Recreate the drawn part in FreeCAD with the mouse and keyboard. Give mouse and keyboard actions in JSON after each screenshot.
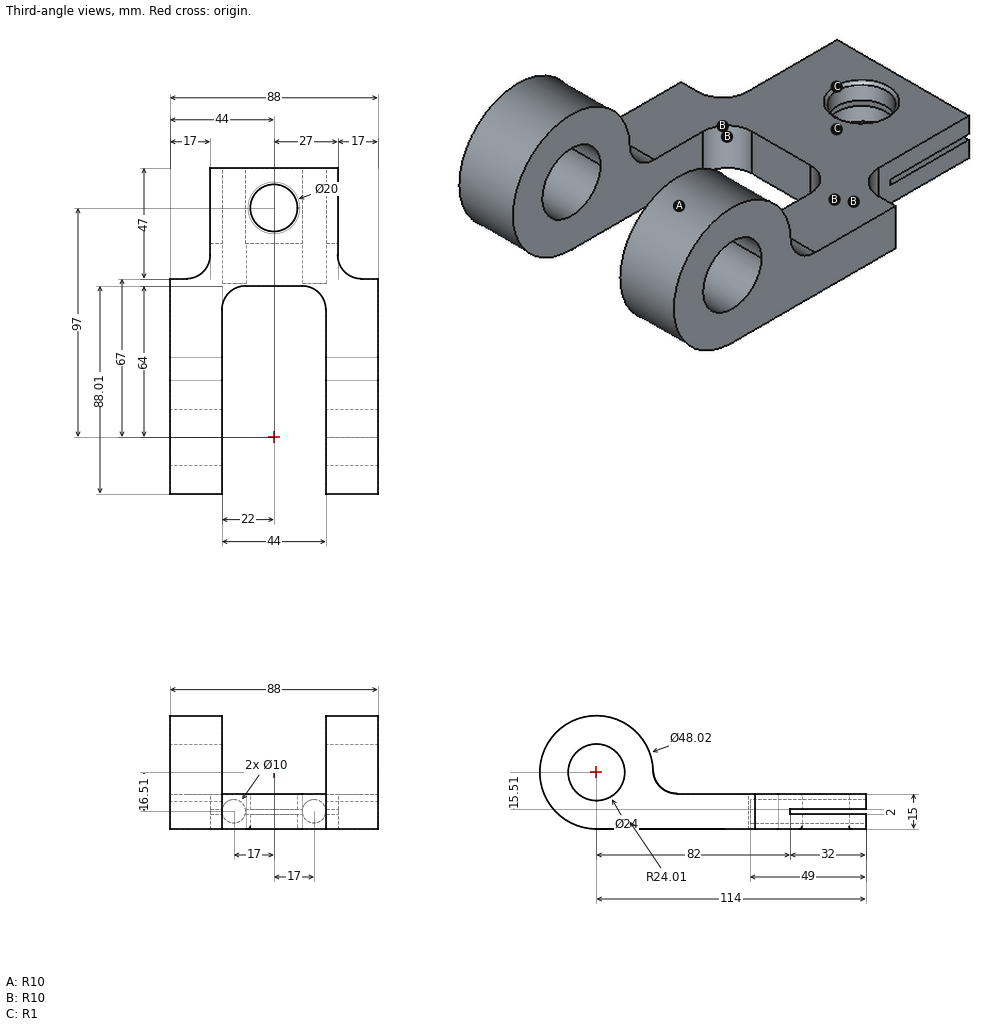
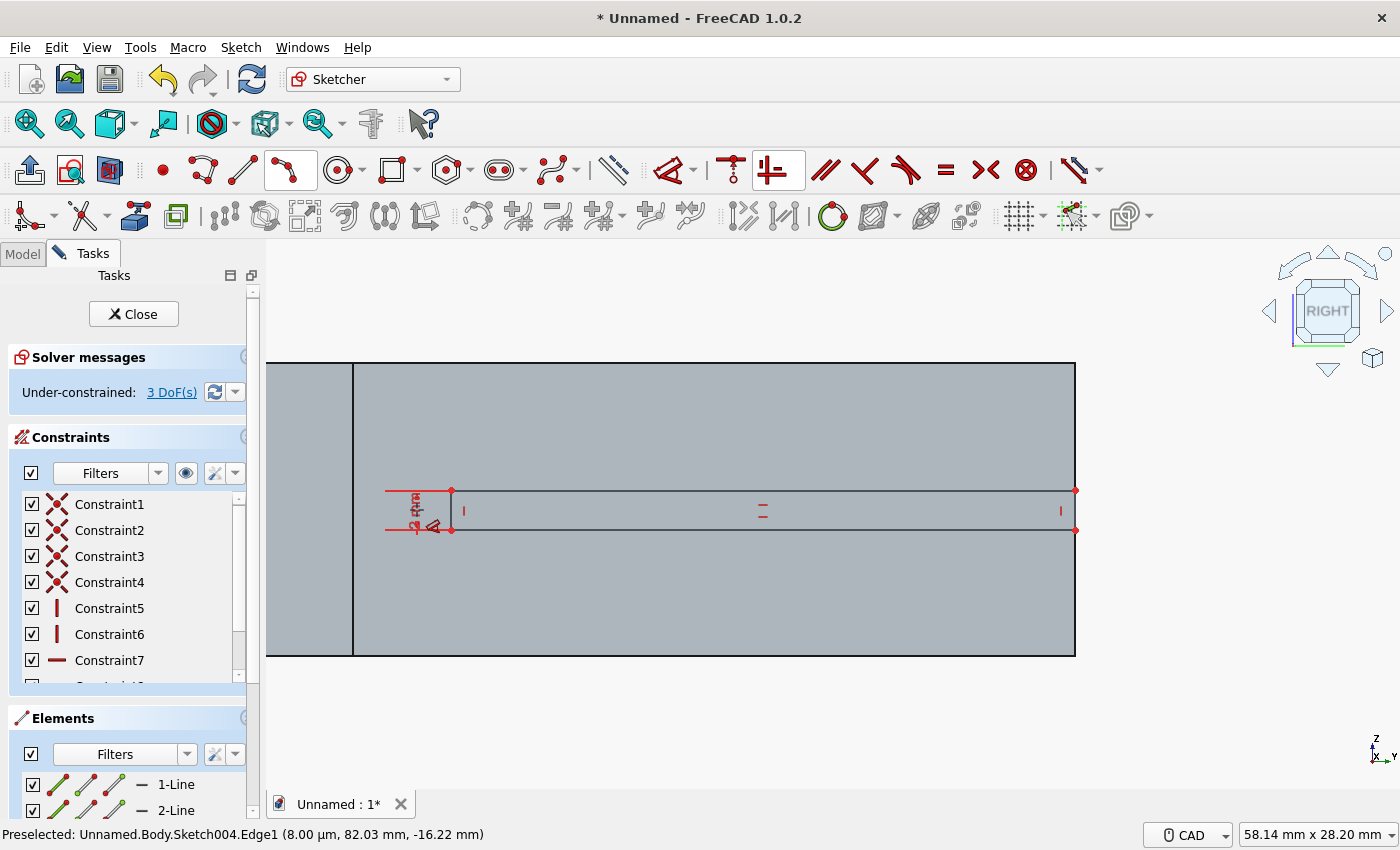
{"action": "left_click", "coordinate": [638, 530]}
{"action": "left_click", "coordinate": [763, 564]}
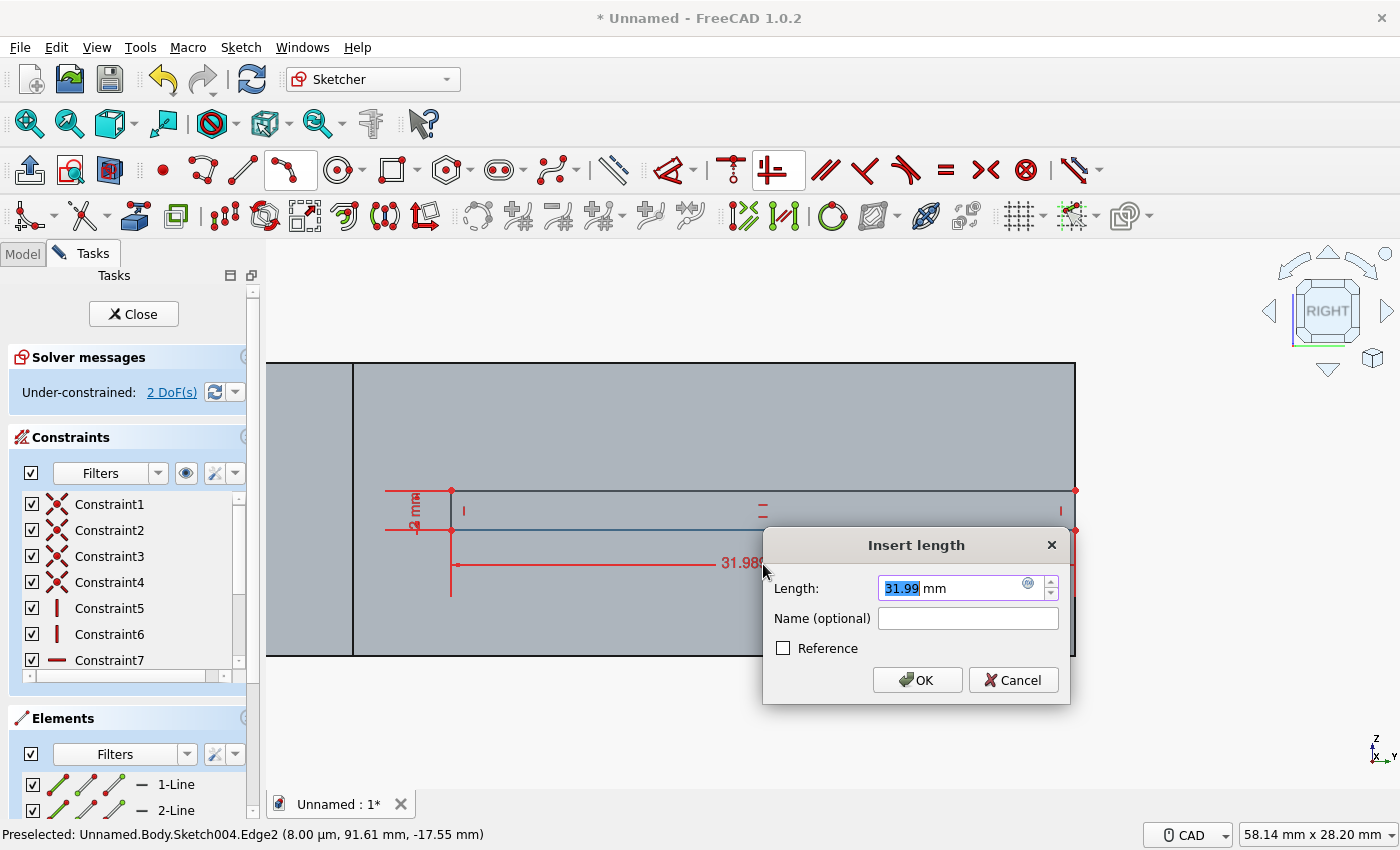
{"action": "type", "text": "32"}
{"action": "key", "text": "Return"}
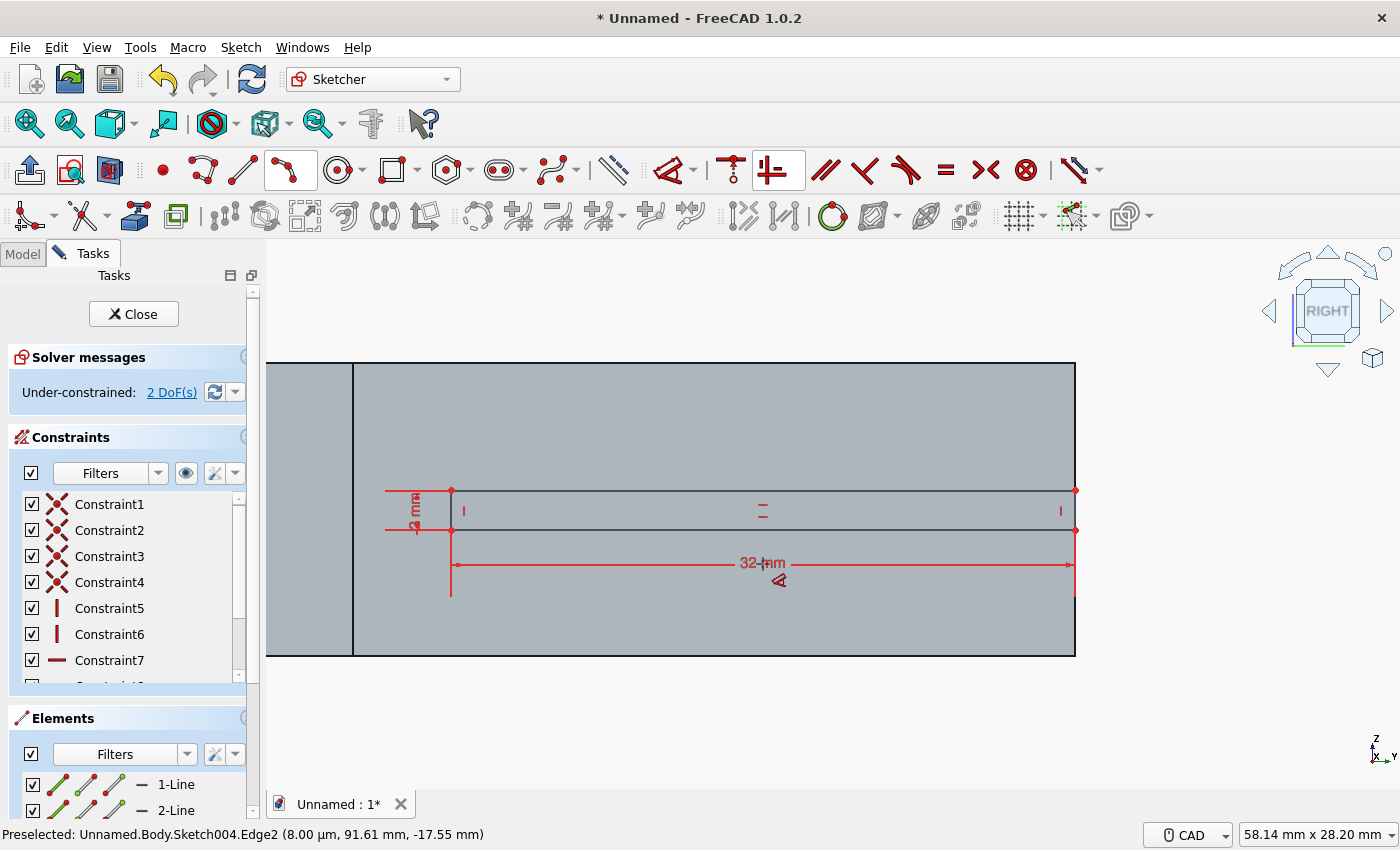
{"action": "left_click", "coordinate": [451, 491]}
{"action": "left_click", "coordinate": [336, 525]}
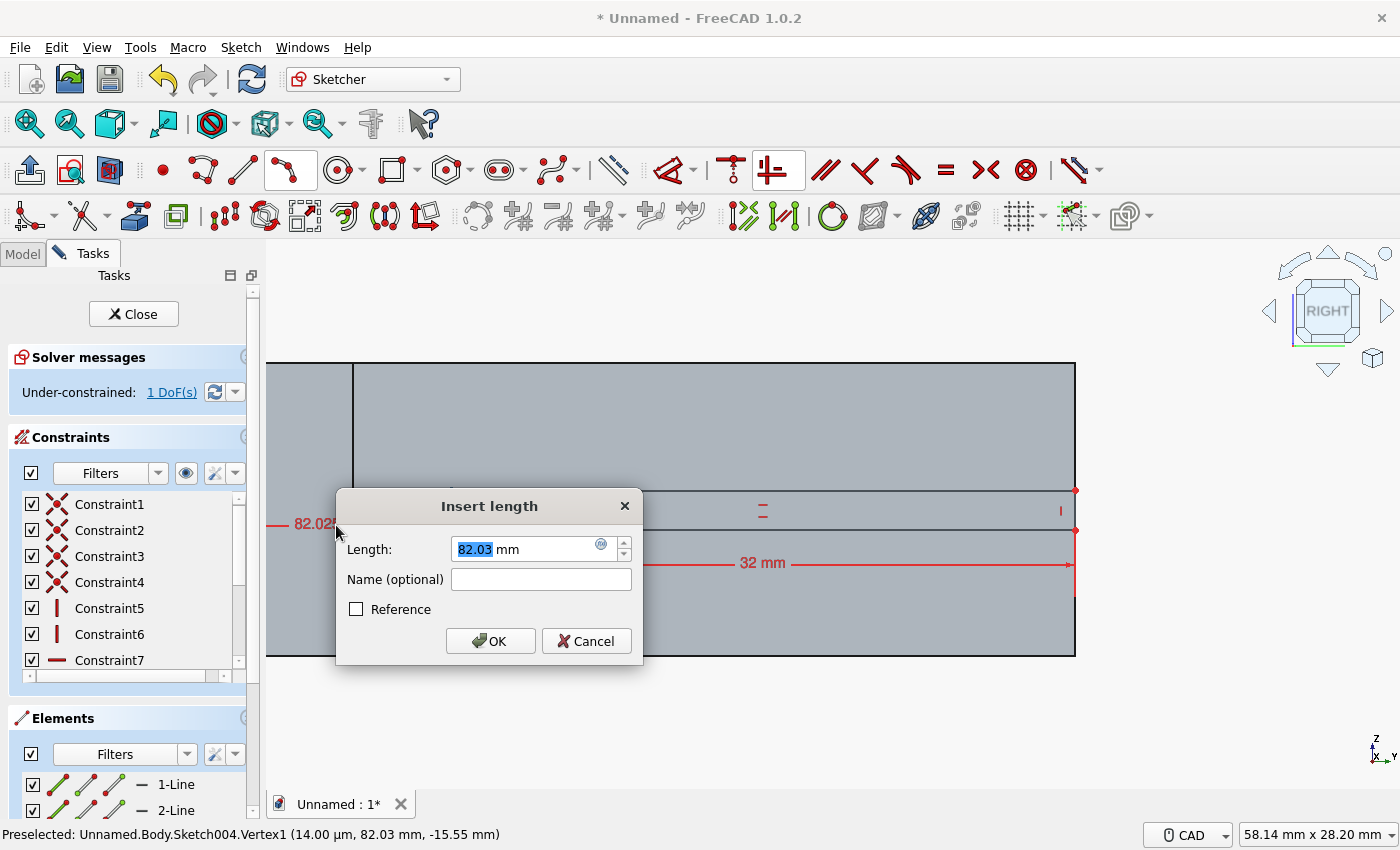
{"action": "type", "text": "82"}
{"action": "key", "text": "Return"}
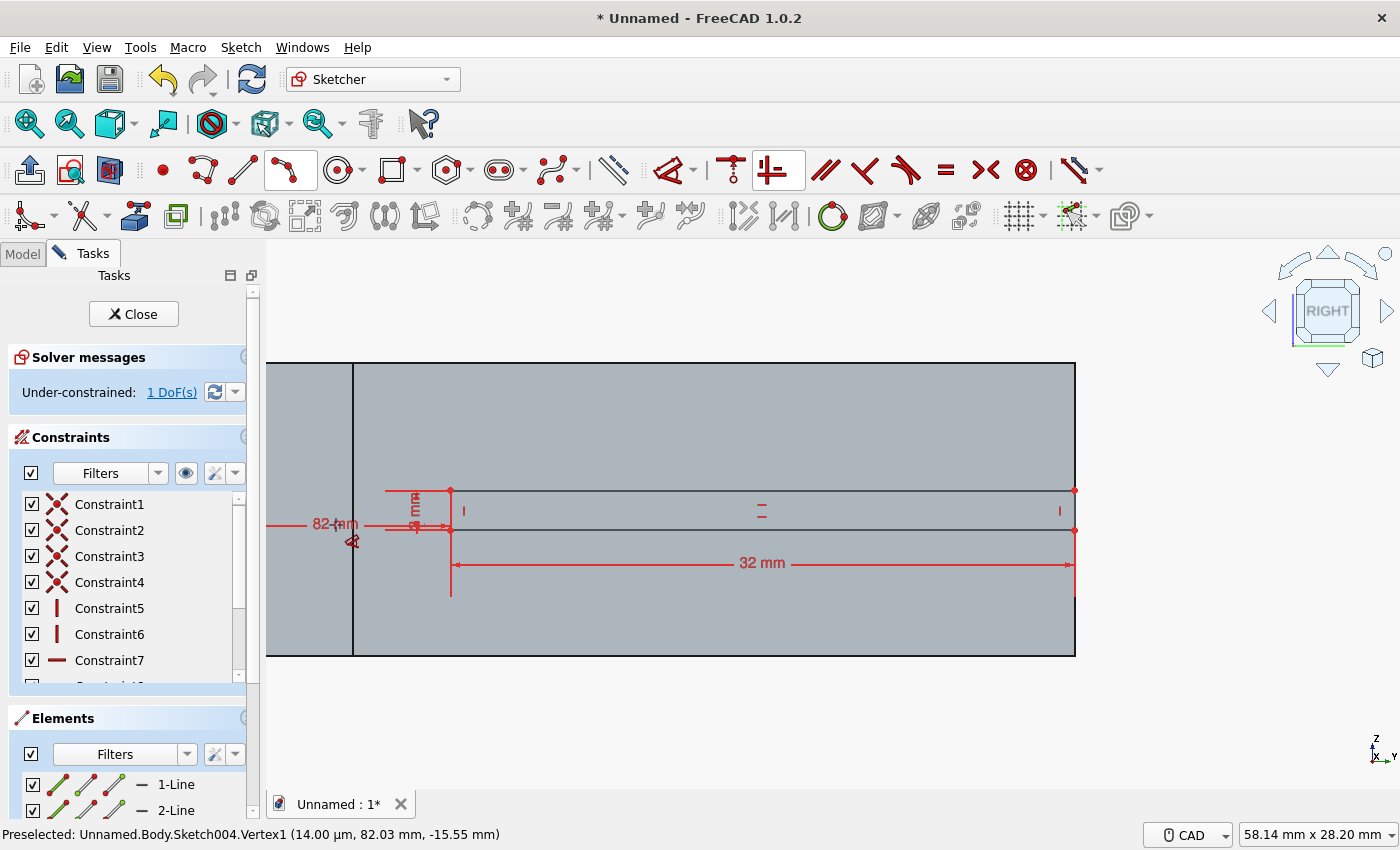
{"action": "left_click", "coordinate": [451, 491]}
{"action": "left_click", "coordinate": [485, 379]}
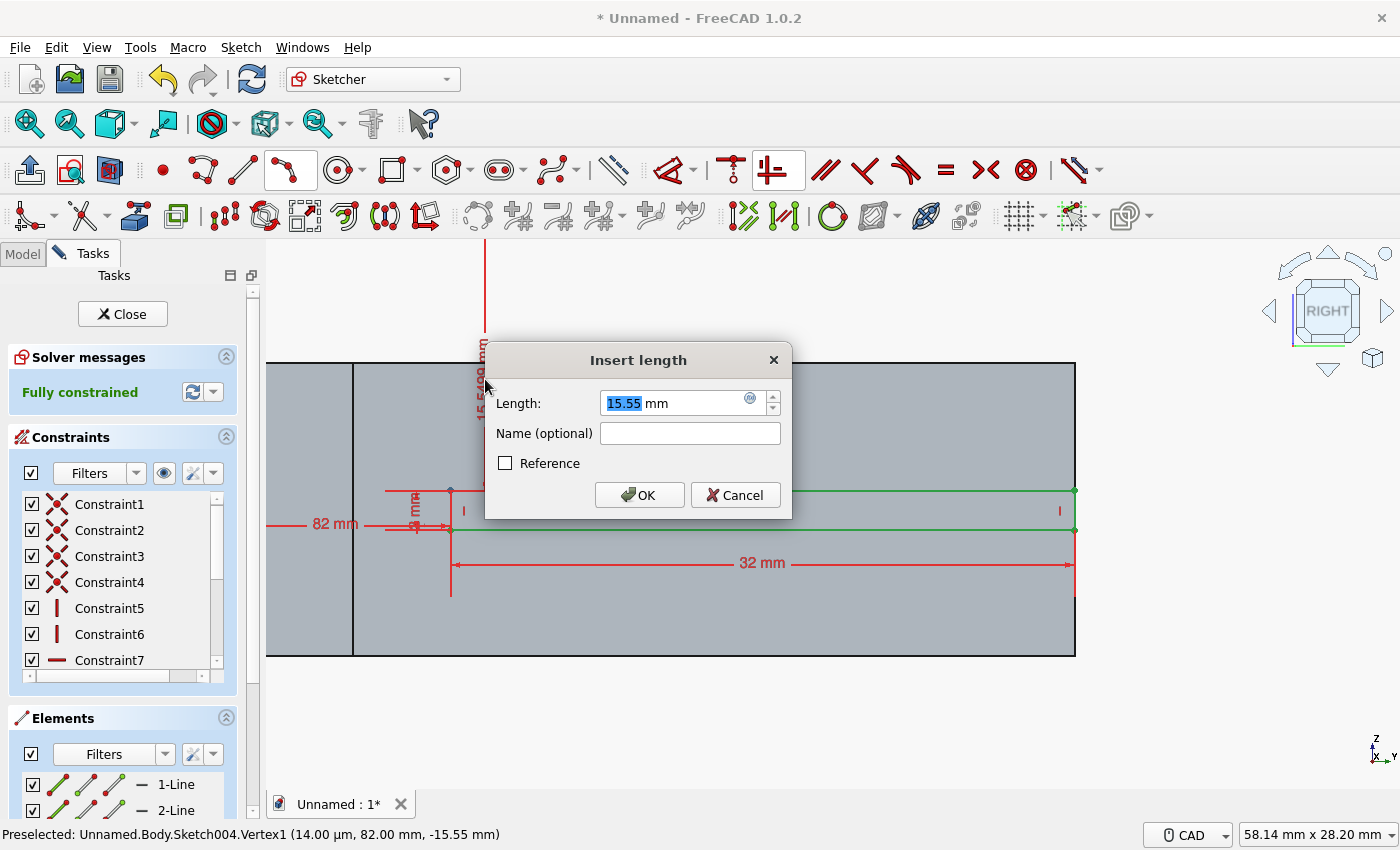
{"action": "type", "text": "15.51"}
{"action": "key", "text": "Return"}
{"action": "key", "text": "Escape"}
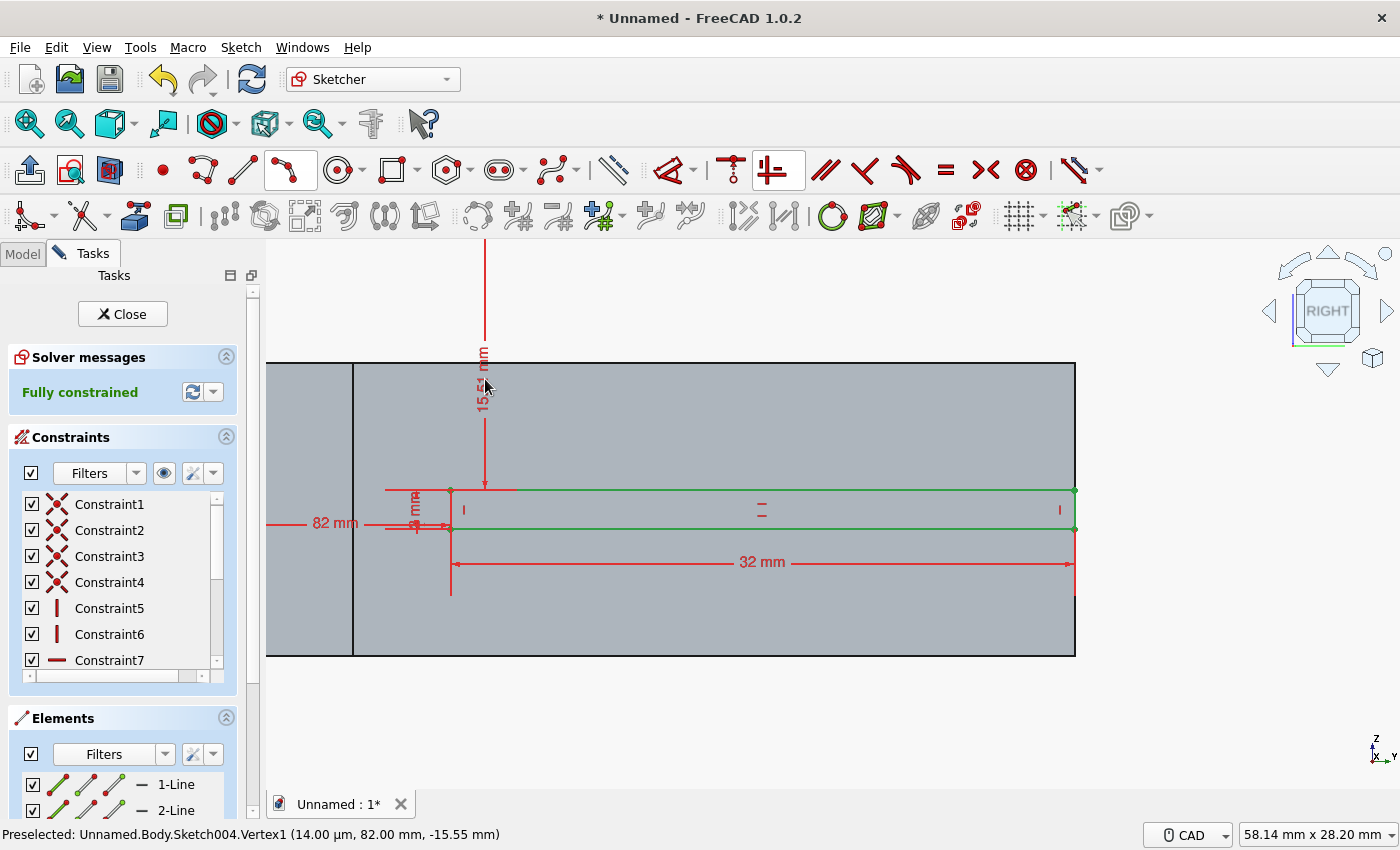
{"action": "left_click", "coordinate": [123, 314]}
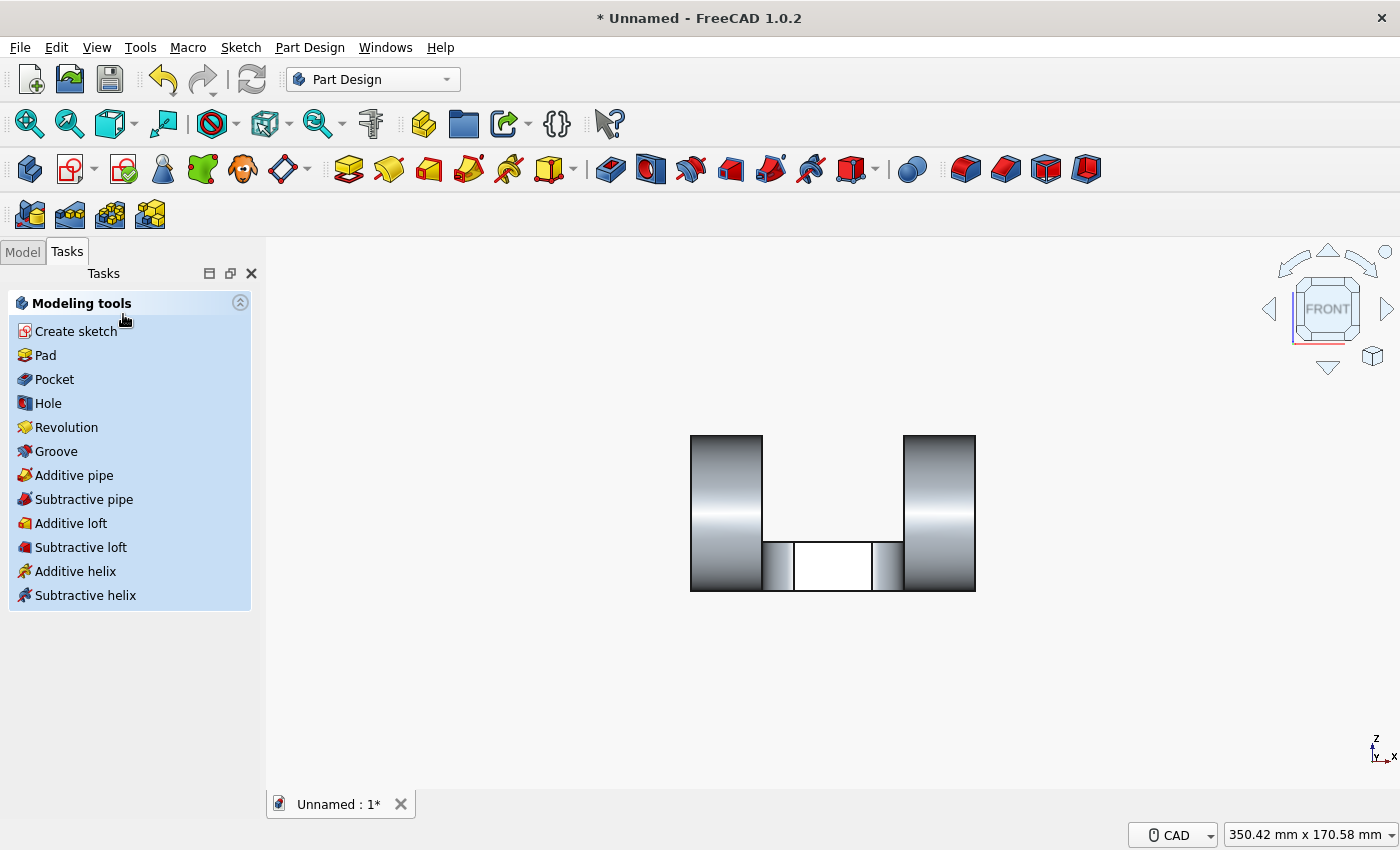
{"action": "left_click", "coordinate": [612, 170]}